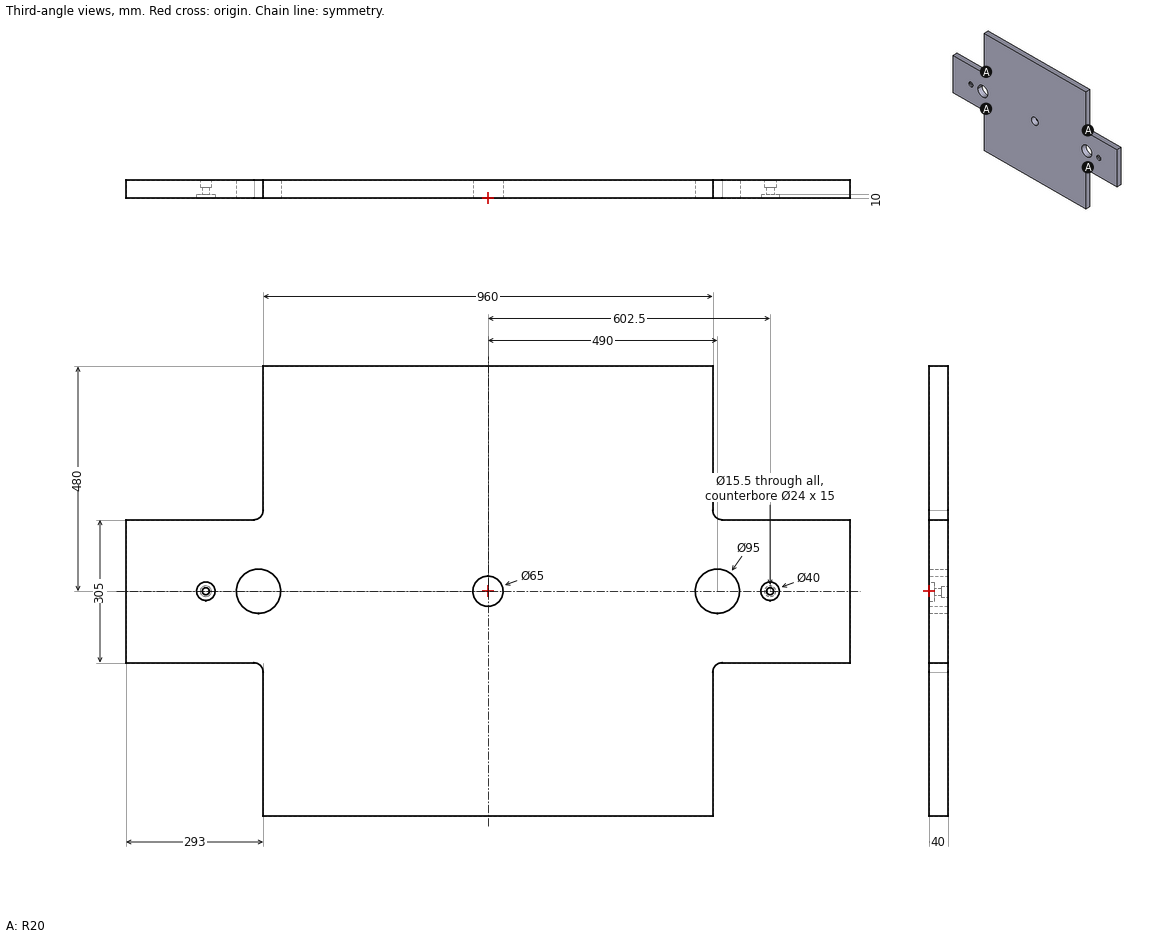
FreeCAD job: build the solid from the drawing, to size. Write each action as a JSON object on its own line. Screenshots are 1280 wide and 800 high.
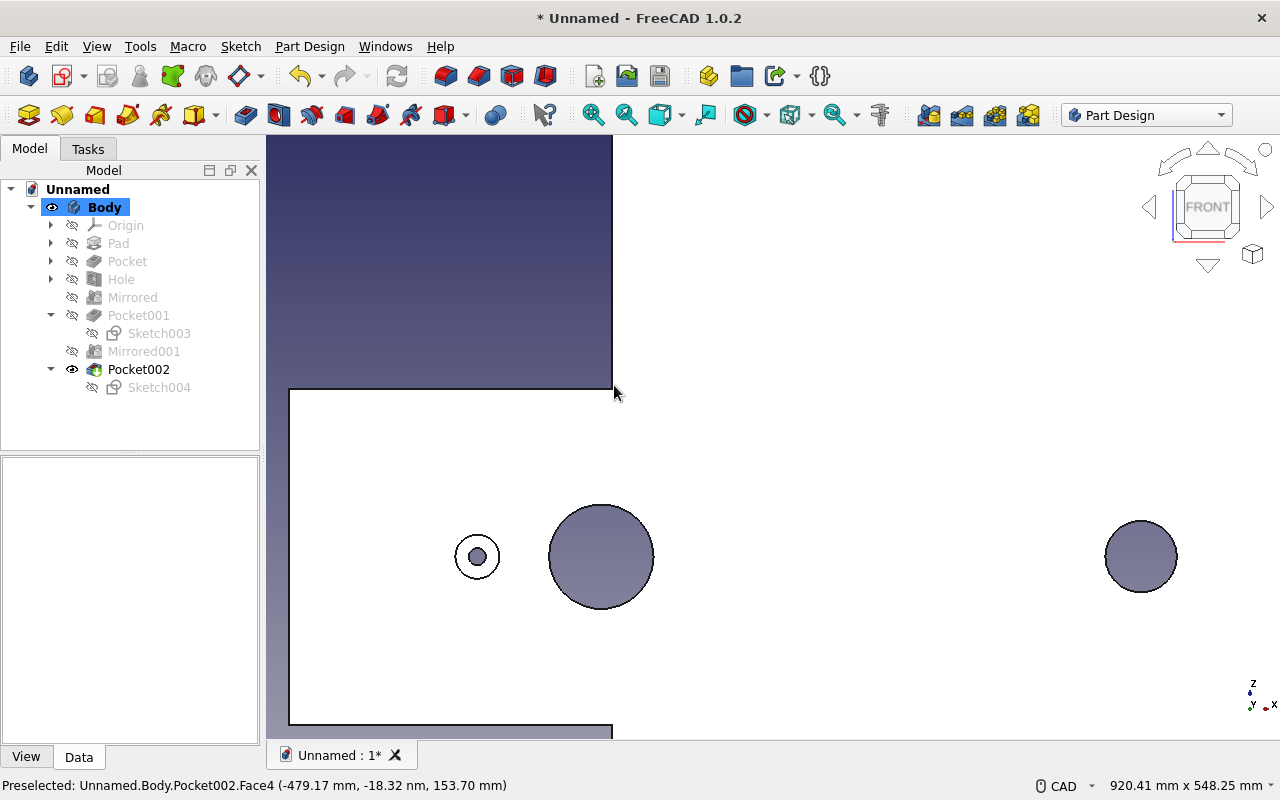
{"action": "key", "text": "v f"}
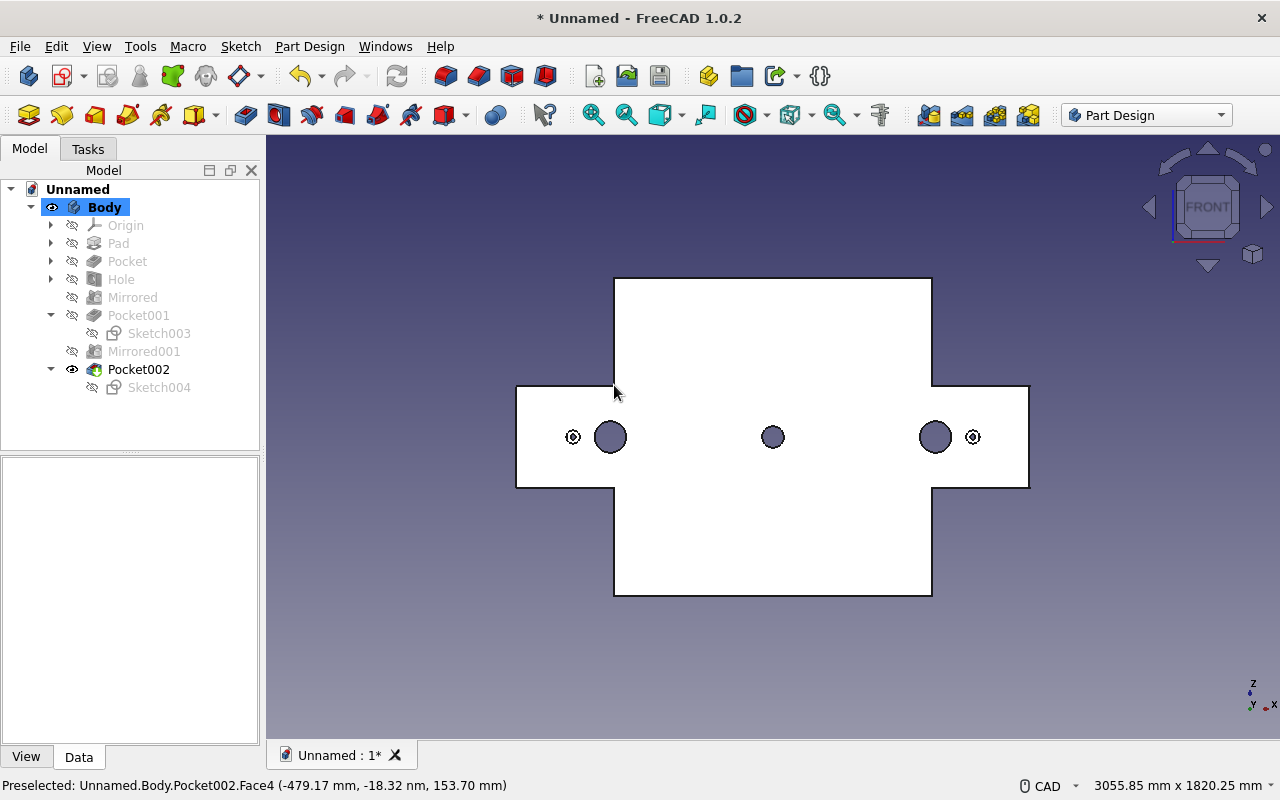
{"action": "key", "text": "3"}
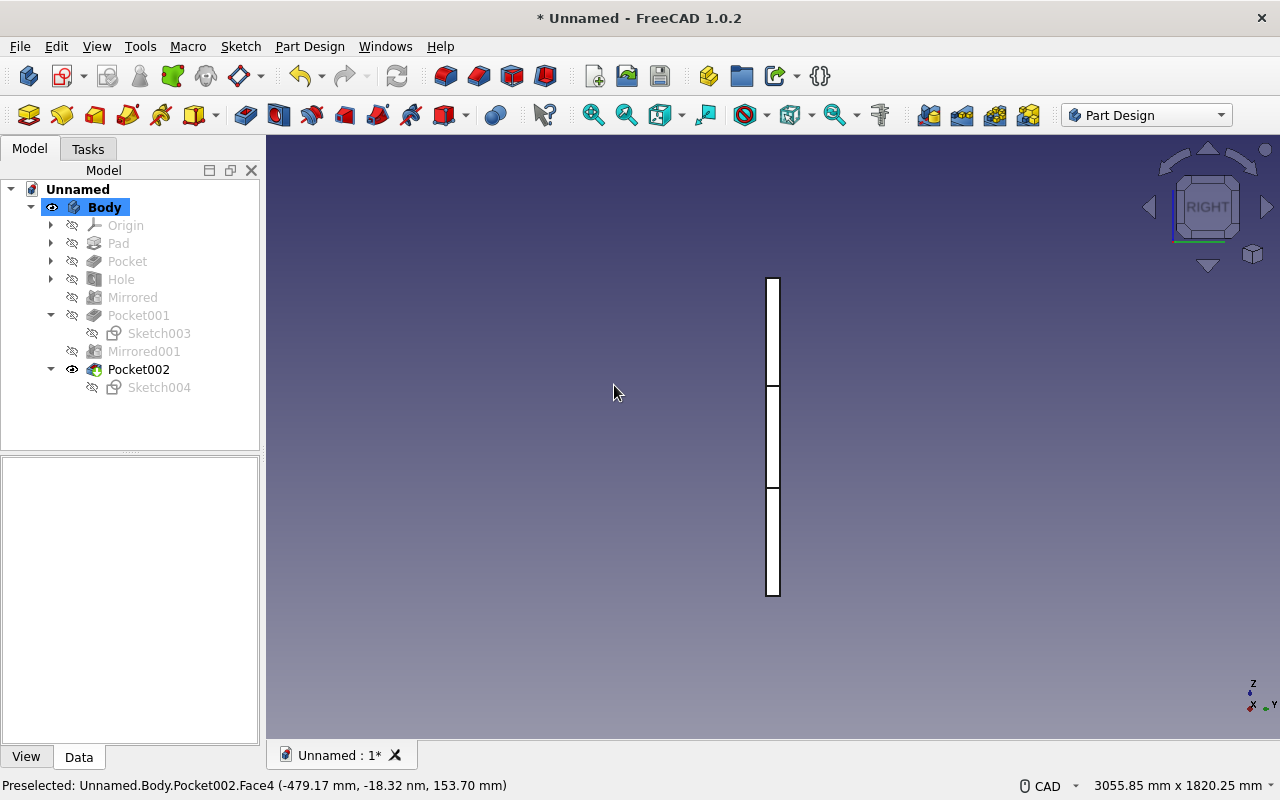
{"action": "scroll", "coordinate": [773, 385], "scroll_direction": "up", "scroll_amount": 6}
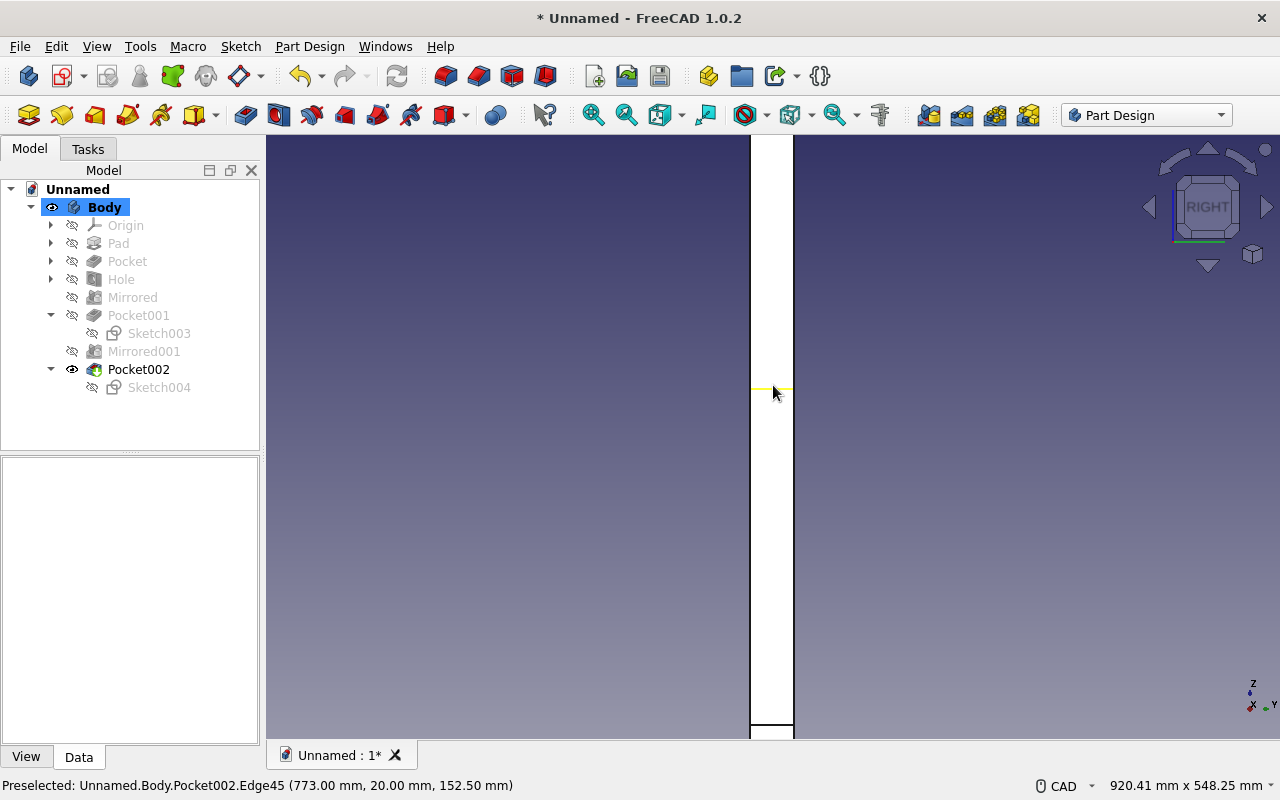
{"action": "key", "text": "v f"}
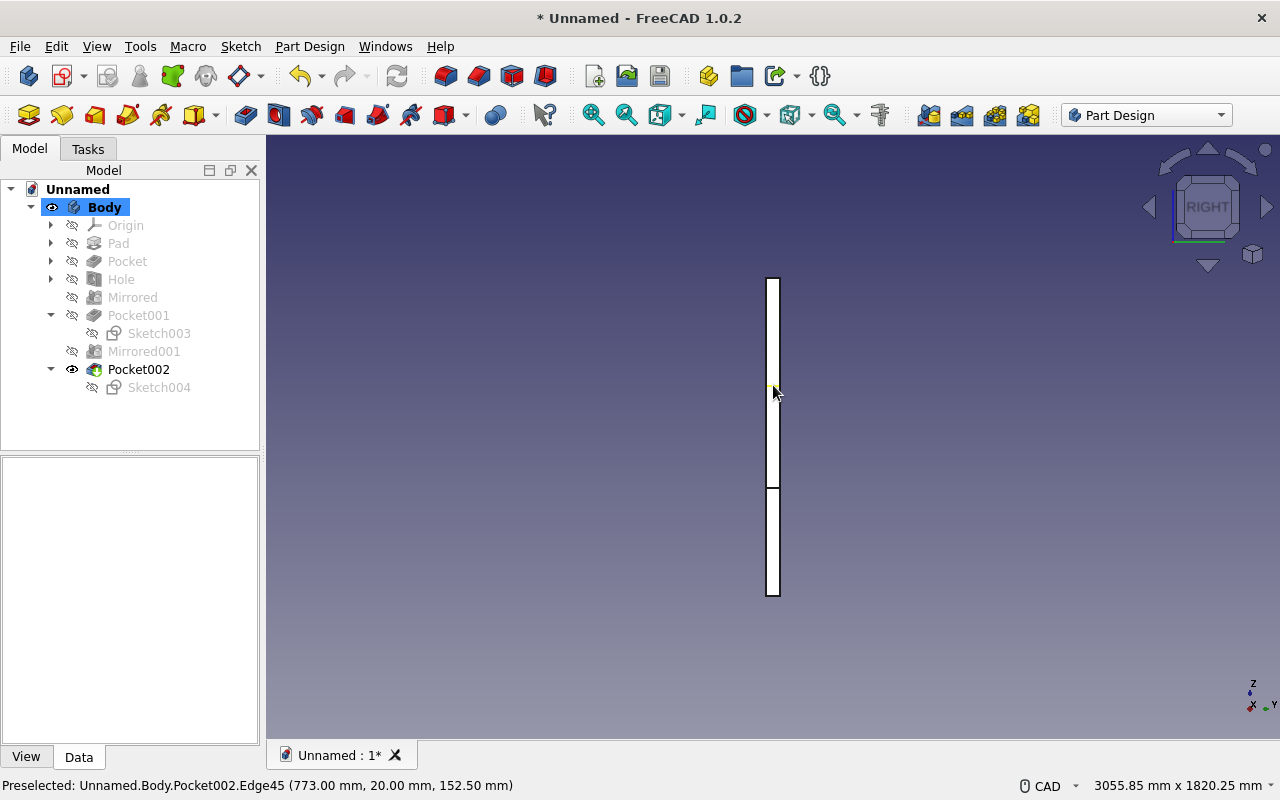
{"action": "key", "text": "5"}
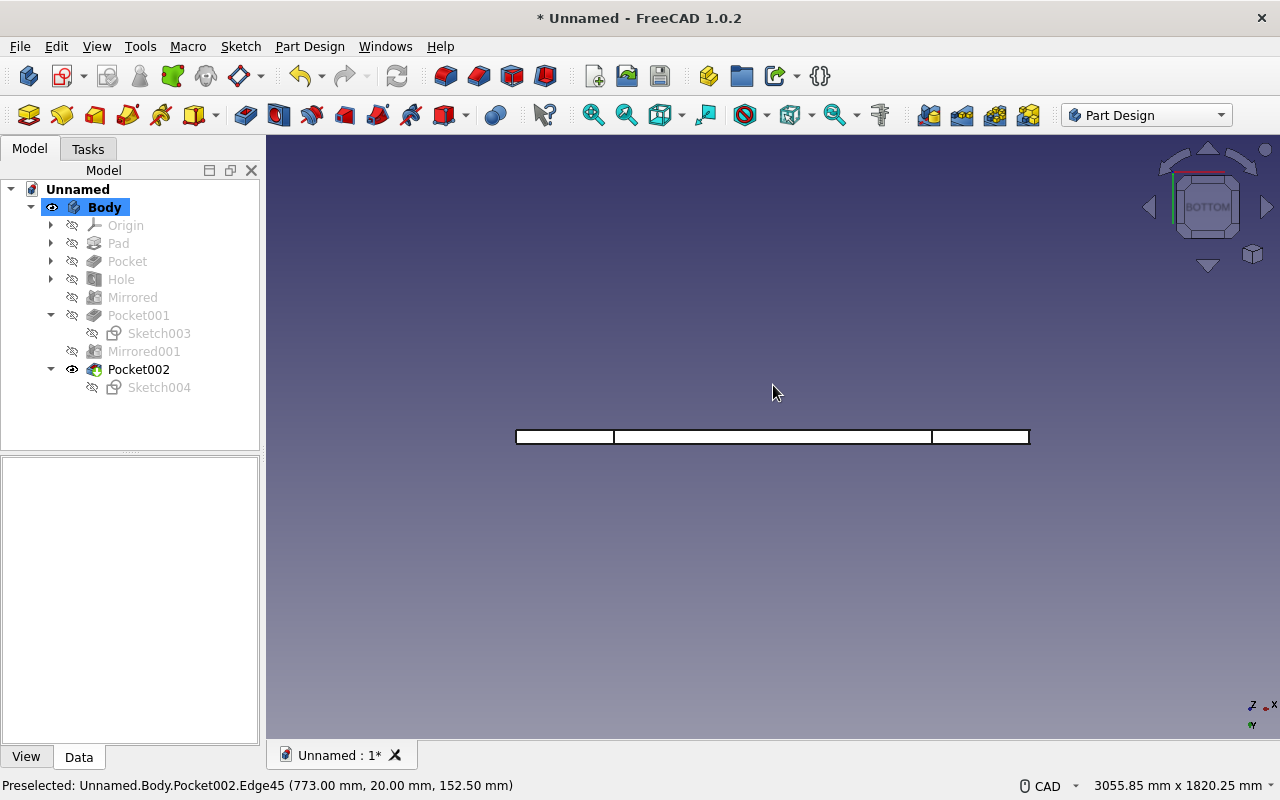
{"action": "scroll", "coordinate": [614, 436], "scroll_direction": "up", "scroll_amount": 6}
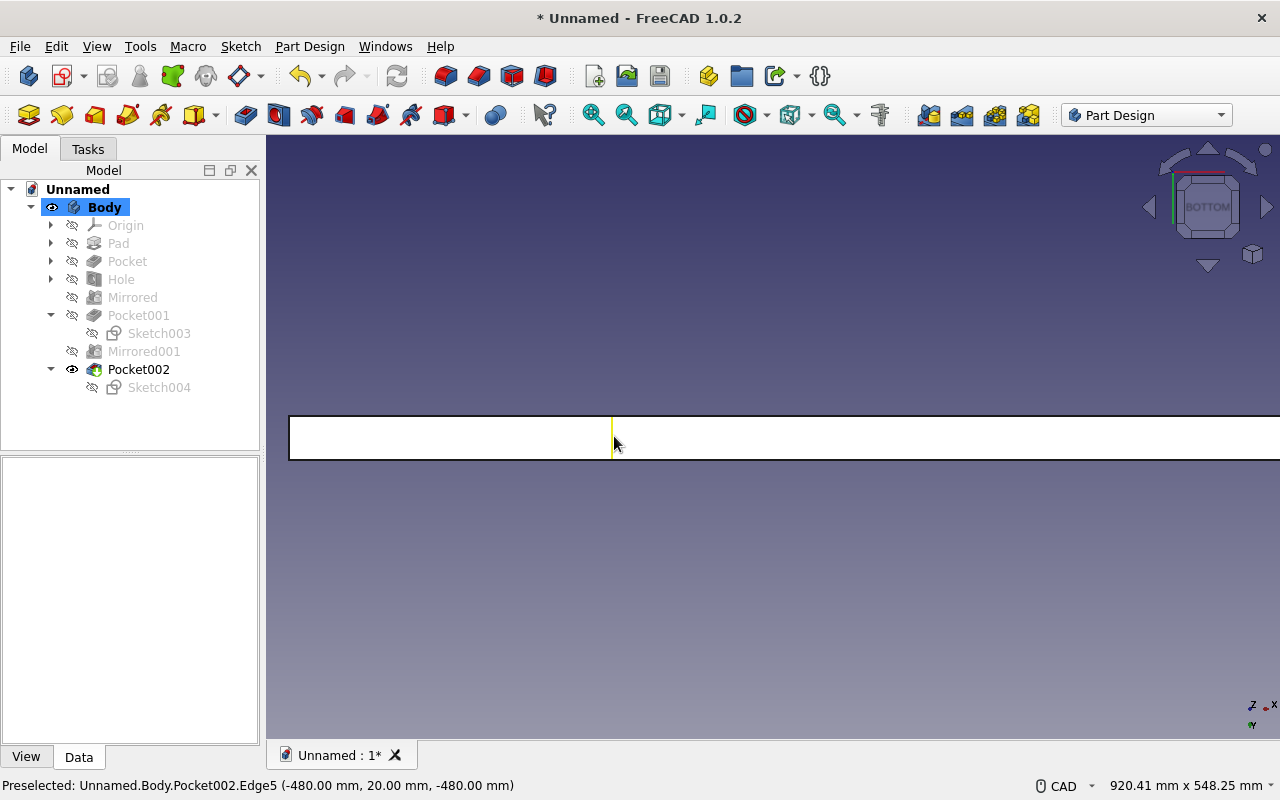
{"action": "key", "text": "v f"}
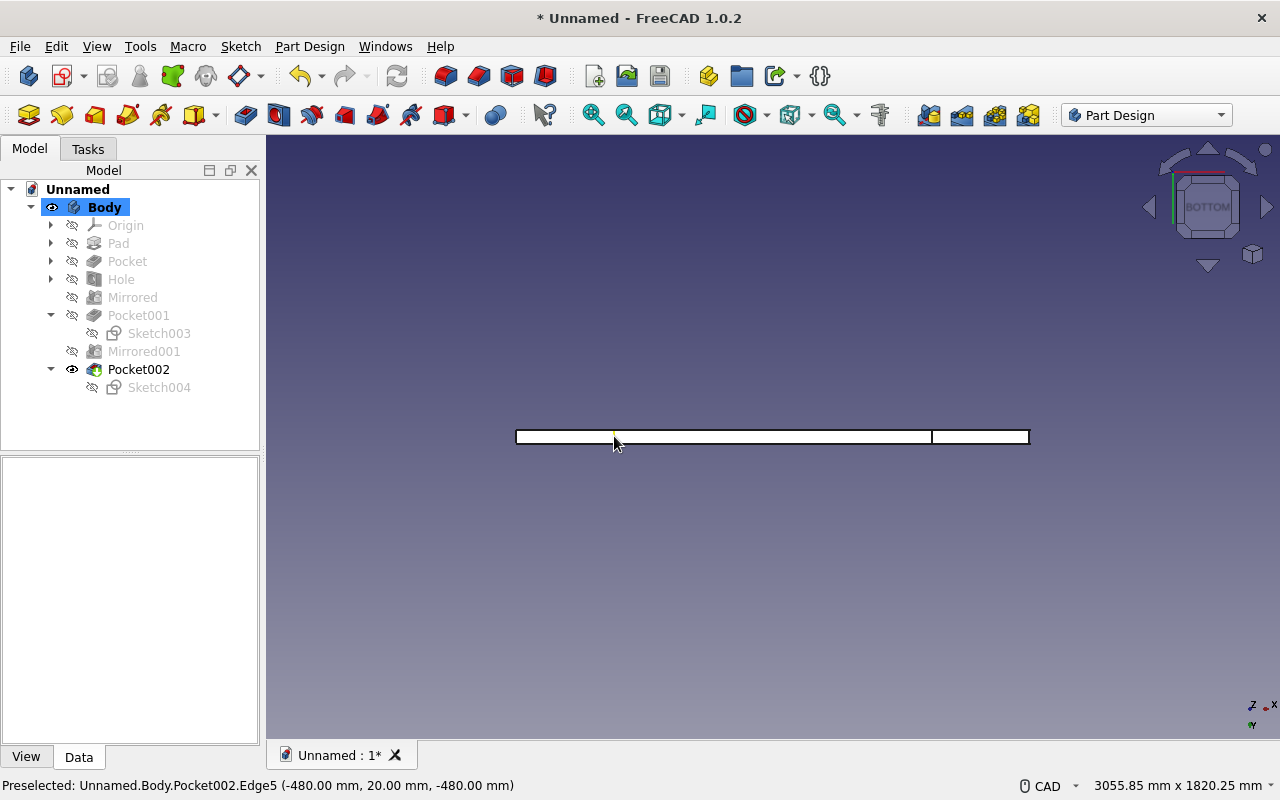
{"action": "key", "text": "4"}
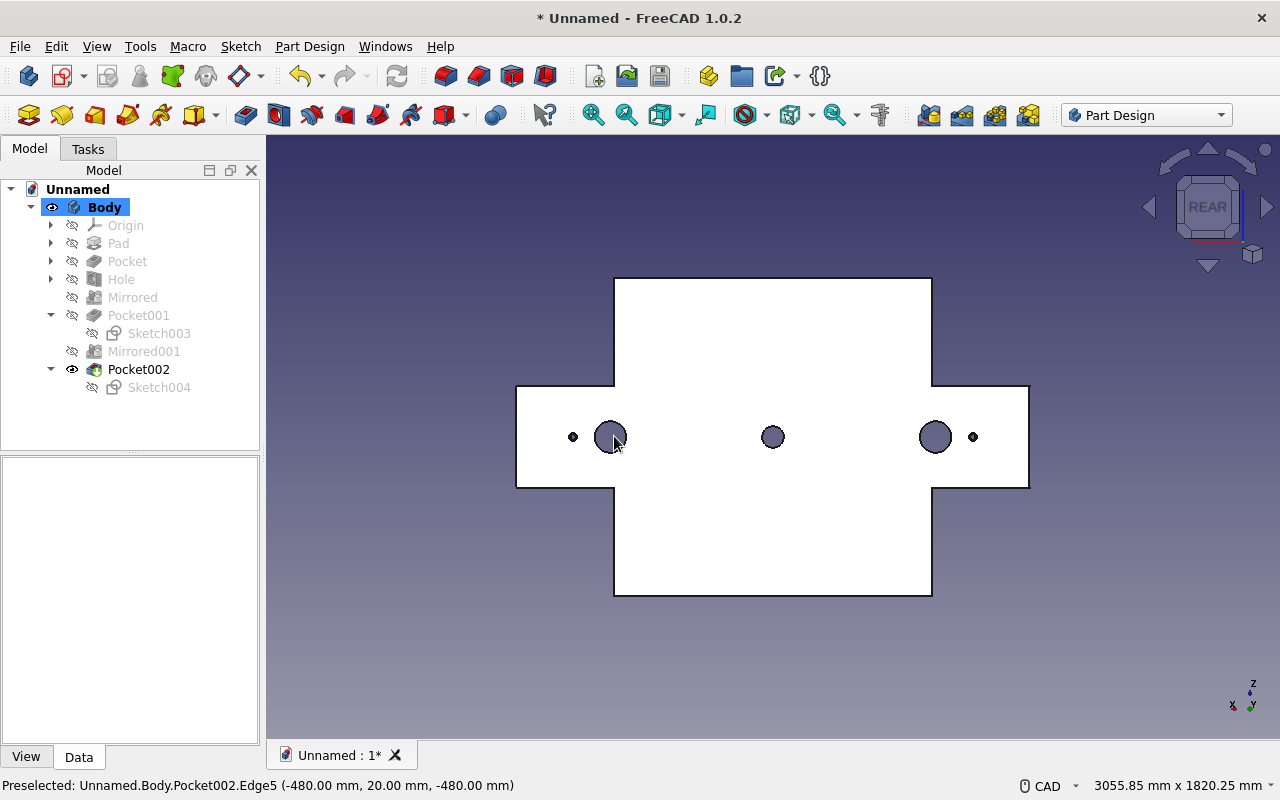
{"action": "scroll", "coordinate": [932, 385], "scroll_direction": "up", "scroll_amount": 6}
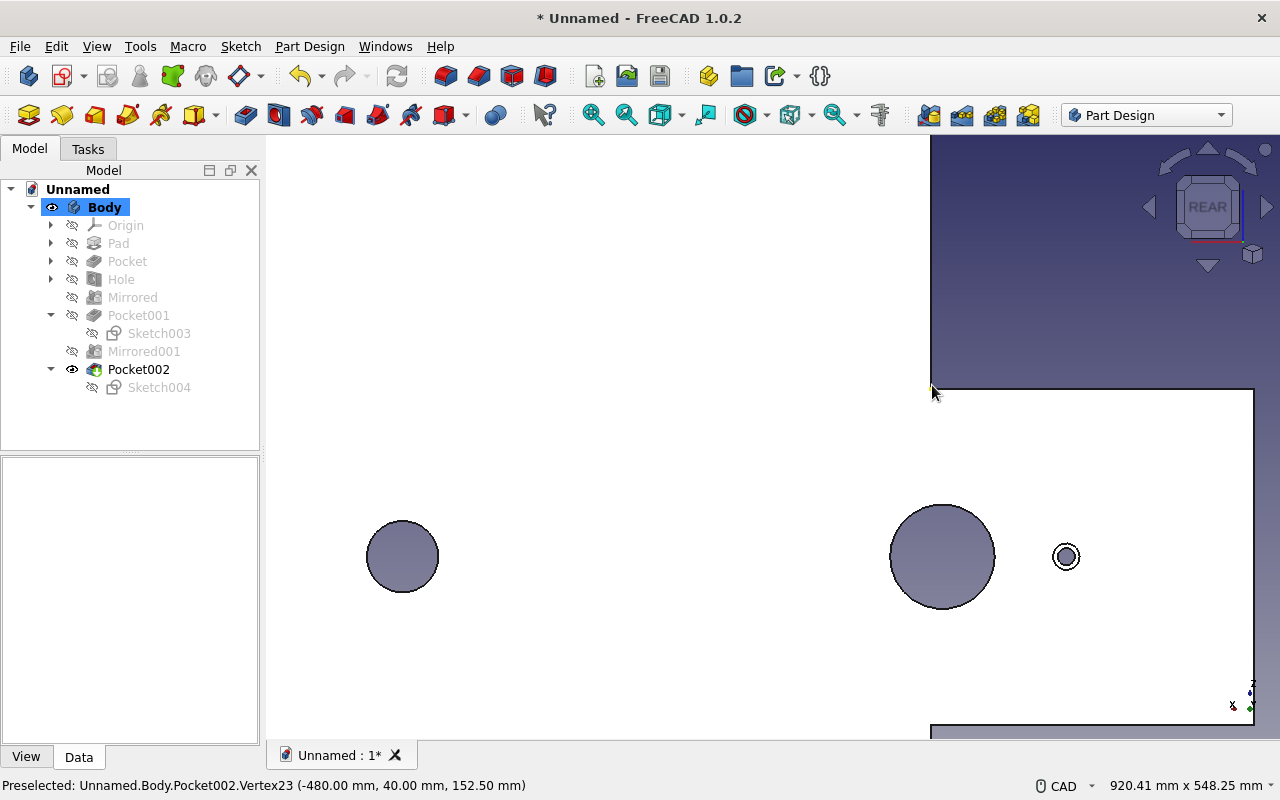
{"action": "key", "text": "v f"}